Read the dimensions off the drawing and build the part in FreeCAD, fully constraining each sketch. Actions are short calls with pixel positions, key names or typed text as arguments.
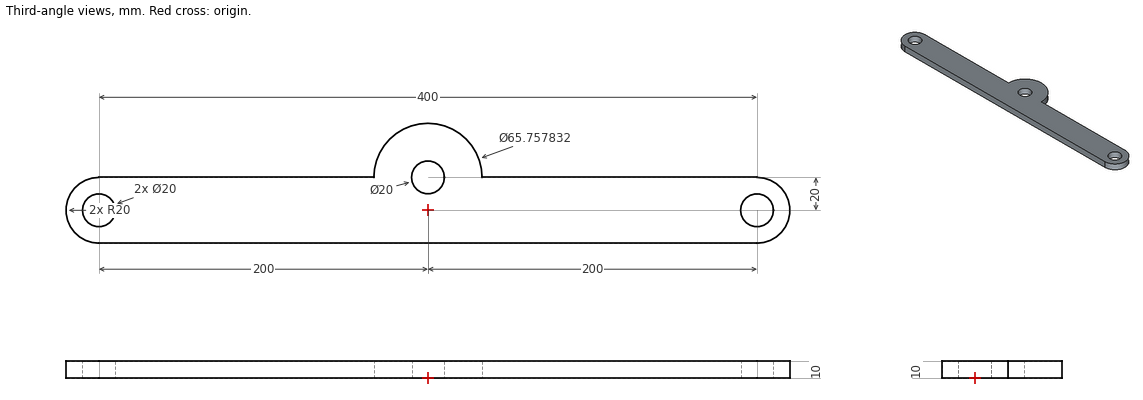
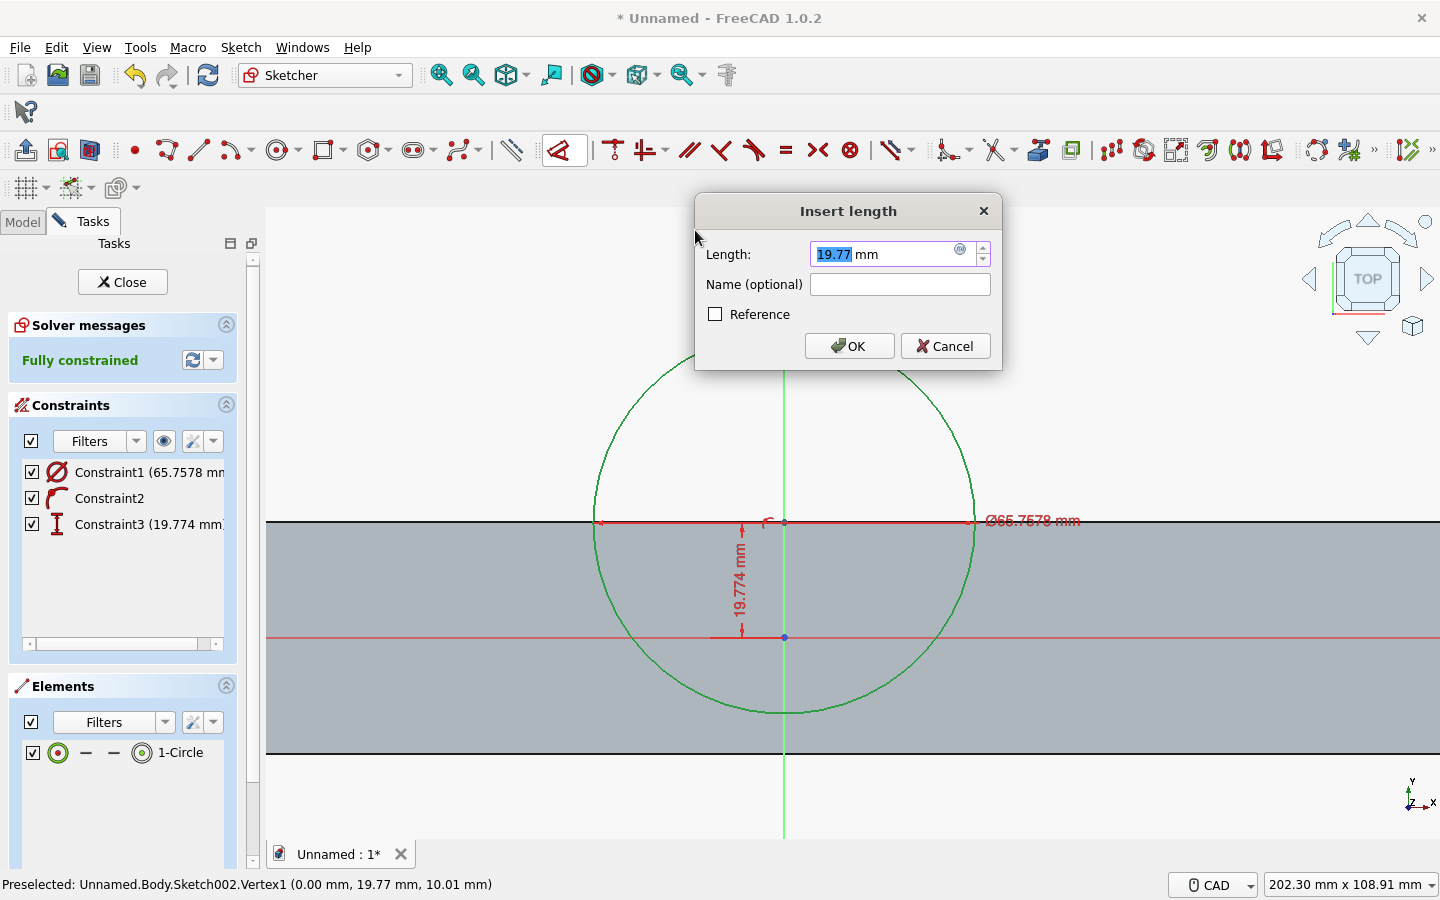
text(20)
key(Return)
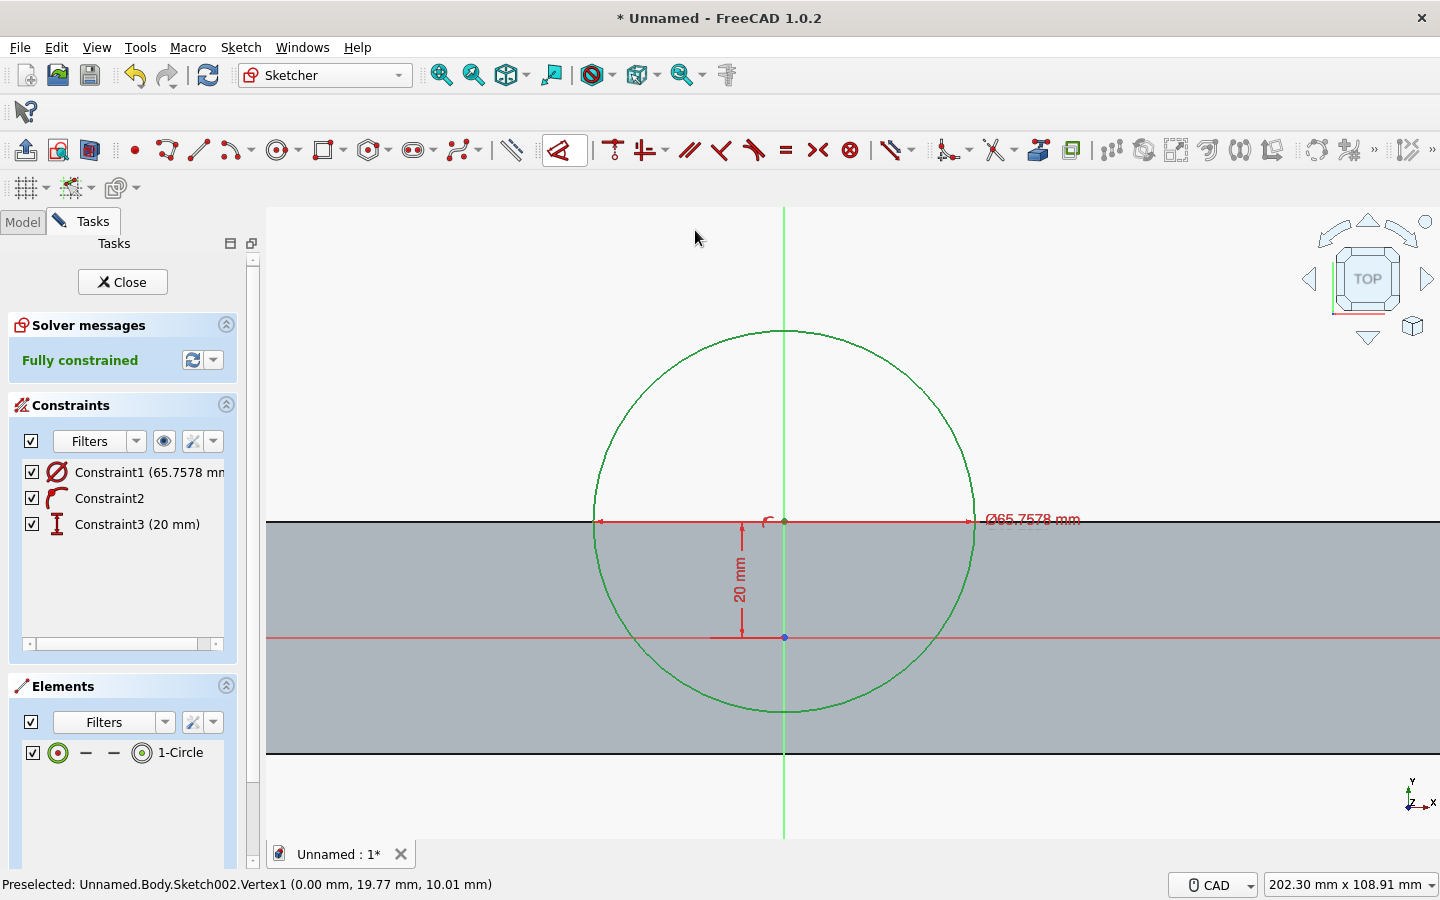
click(123, 282)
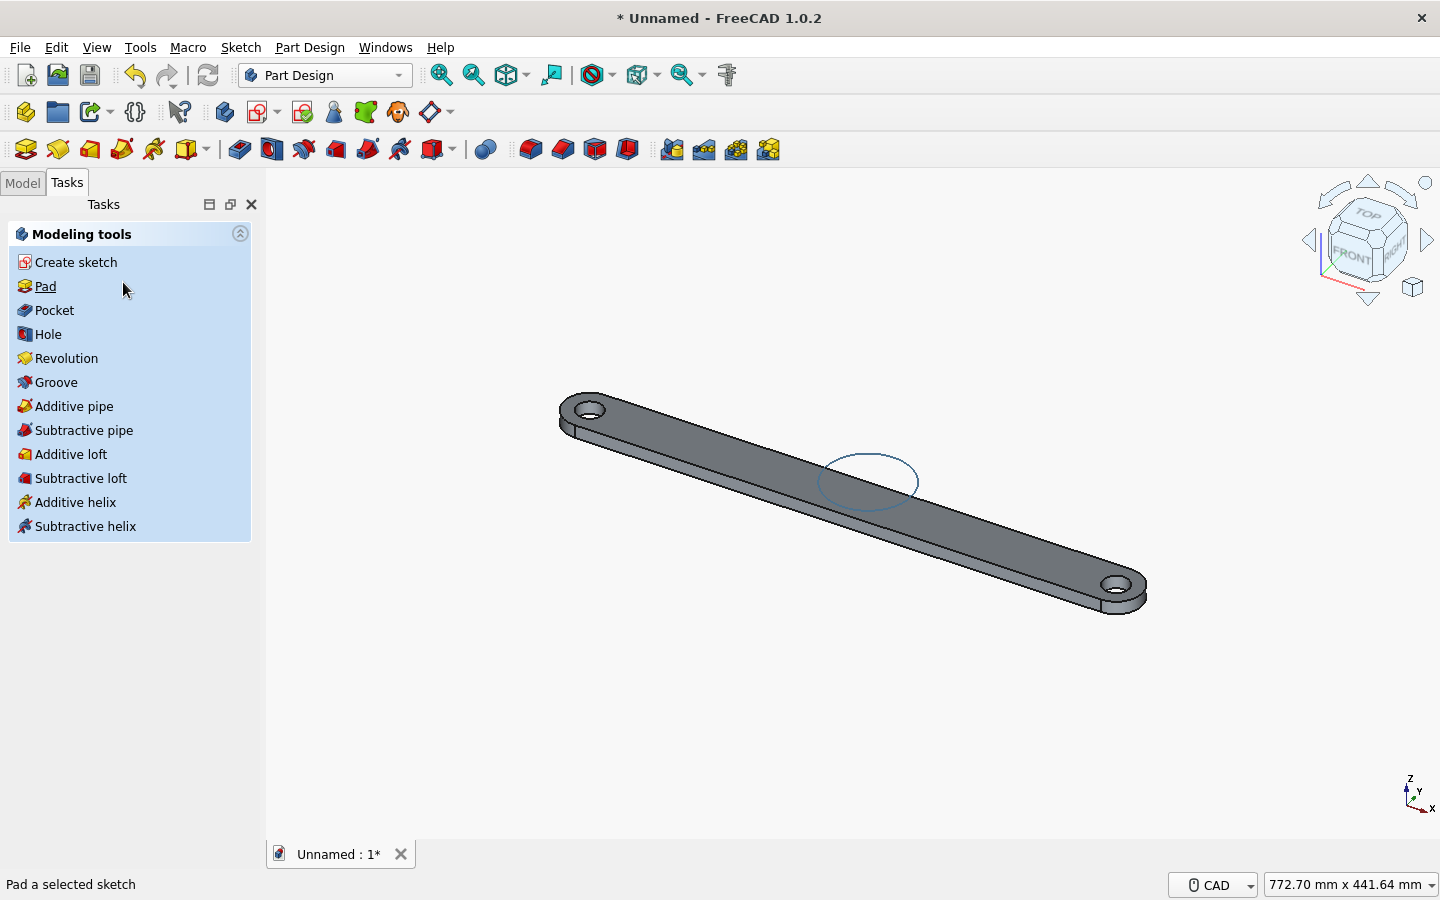
click(26, 150)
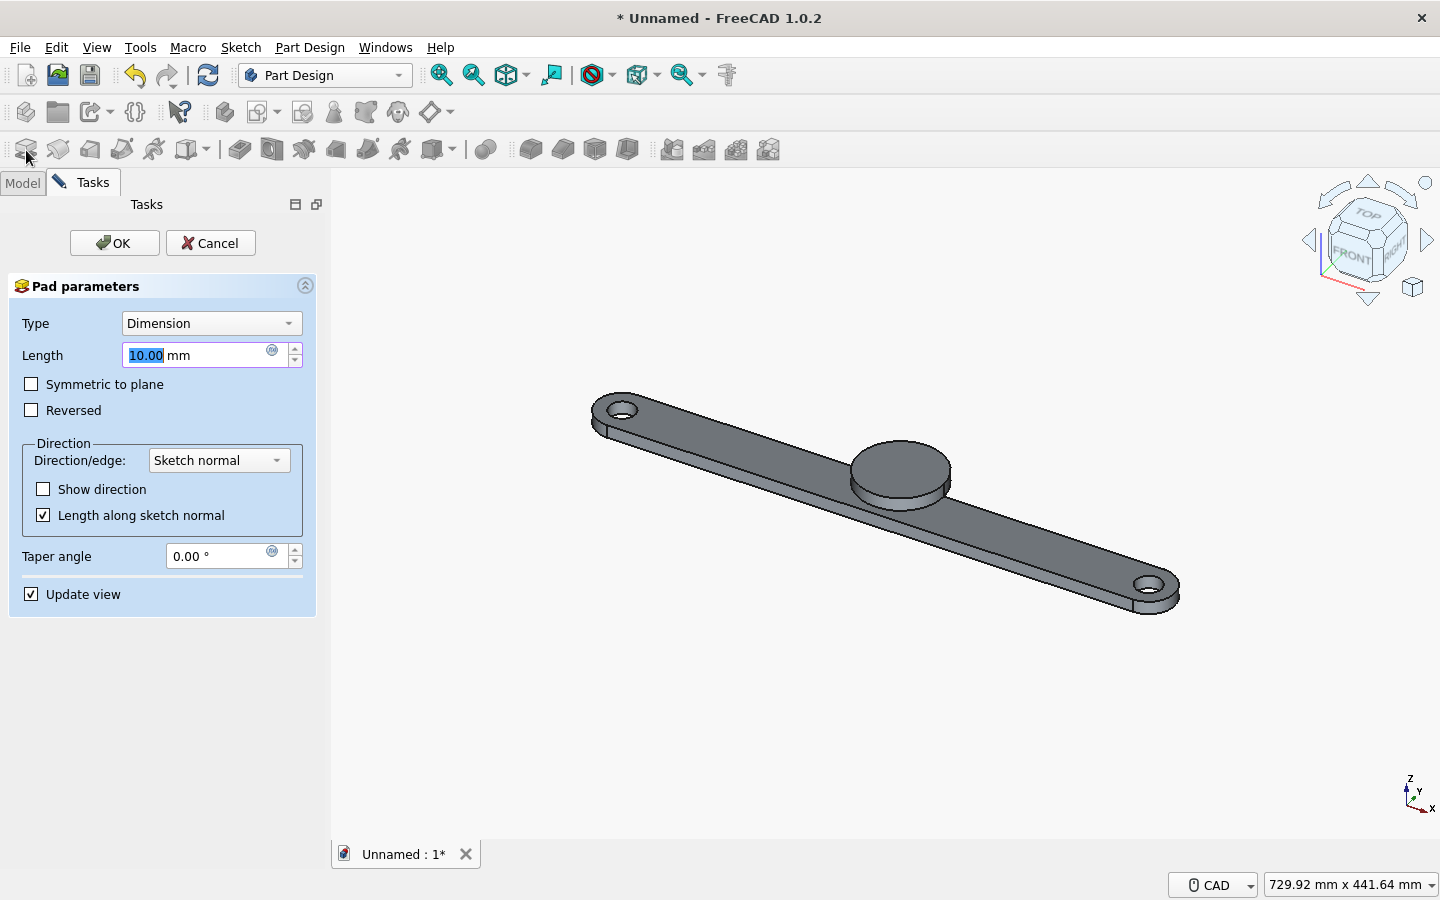
text(10)
key(Tab)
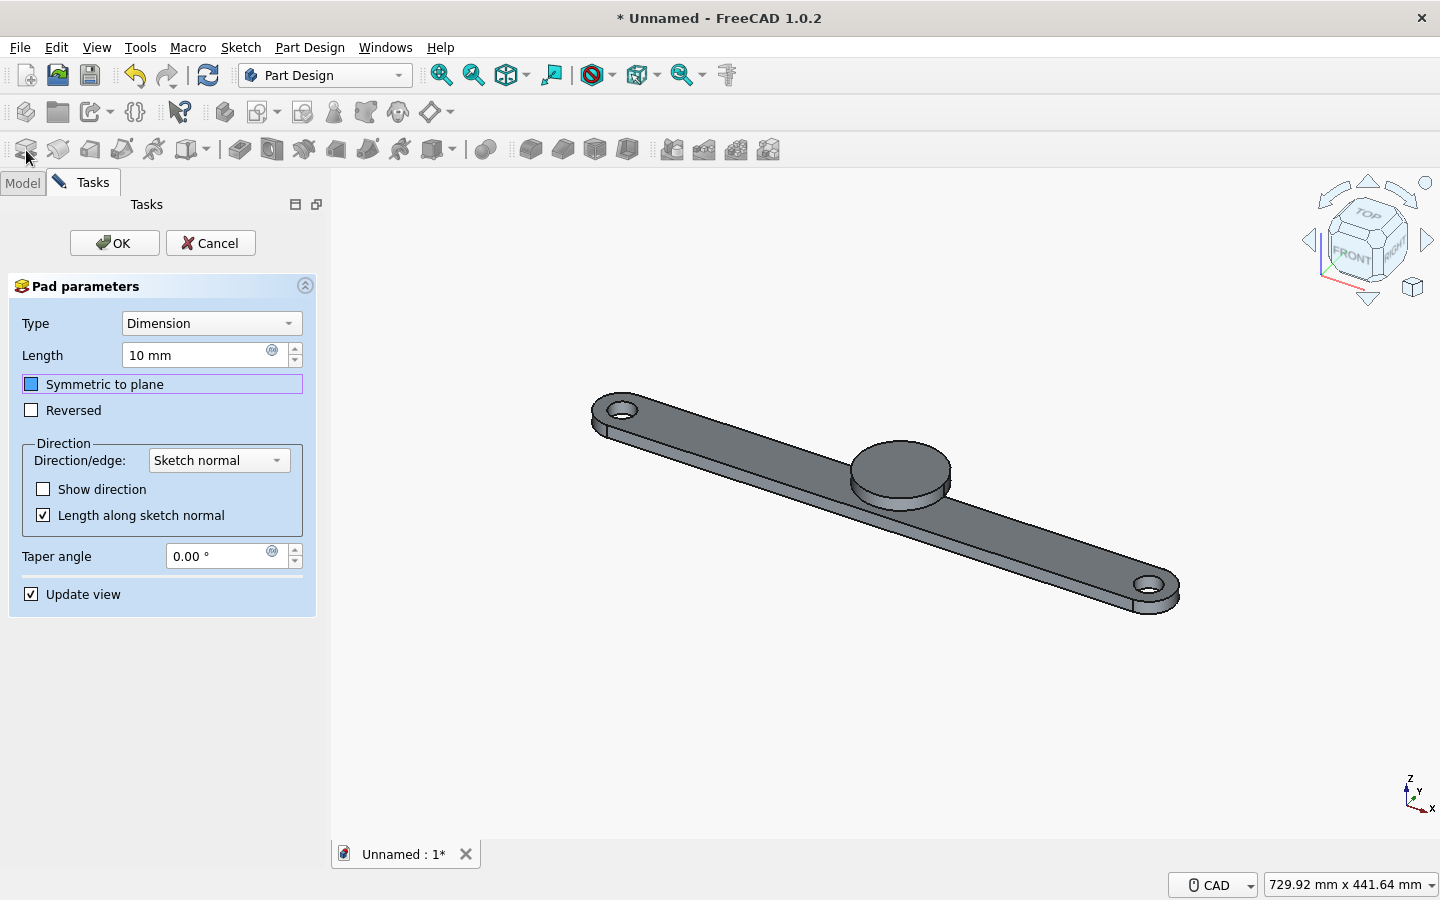
click(30, 410)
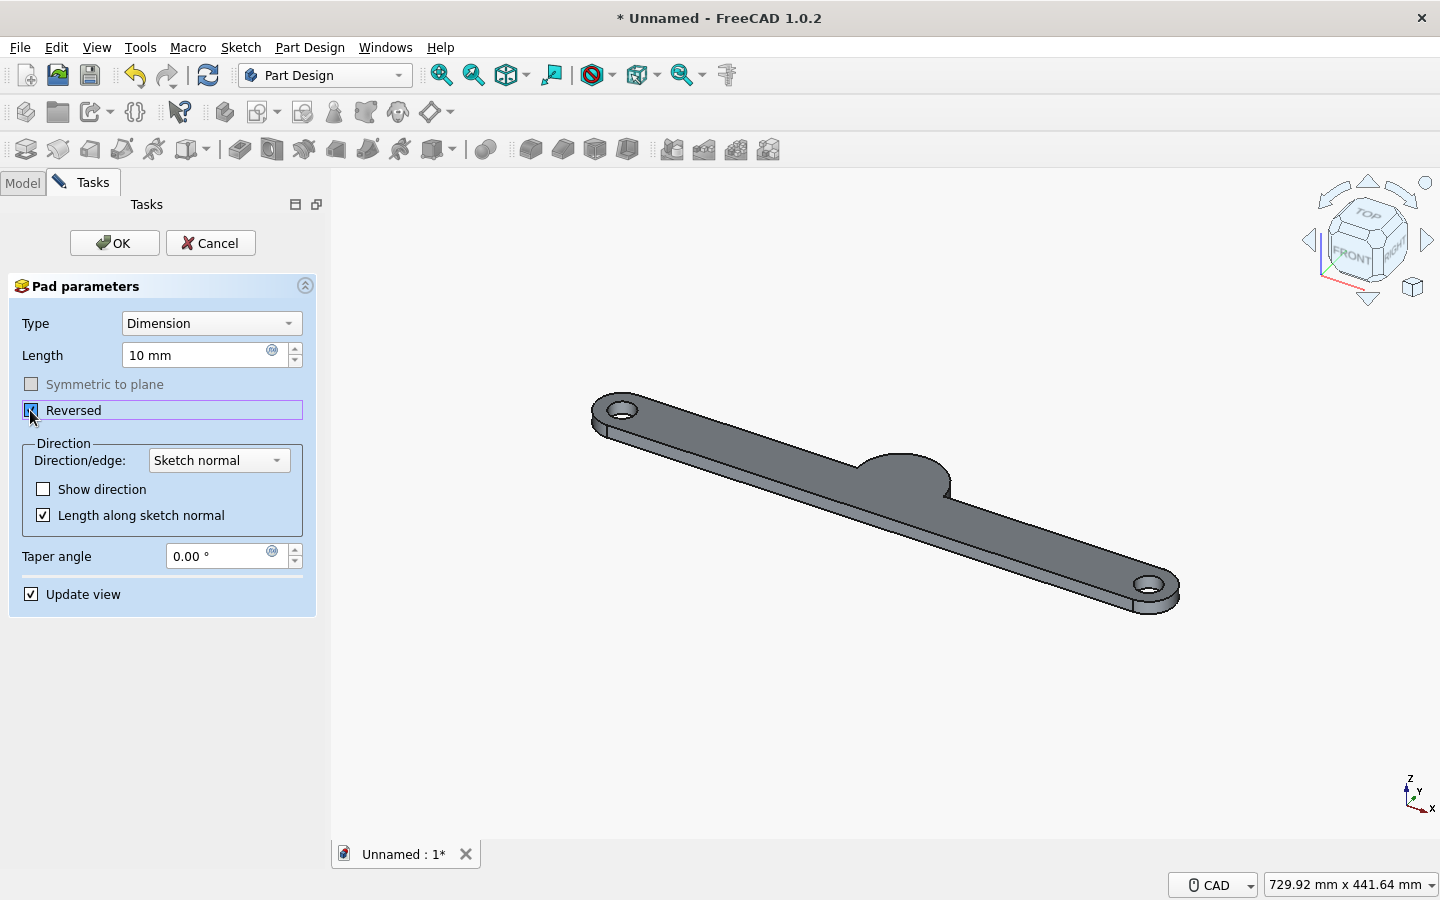
click(115, 243)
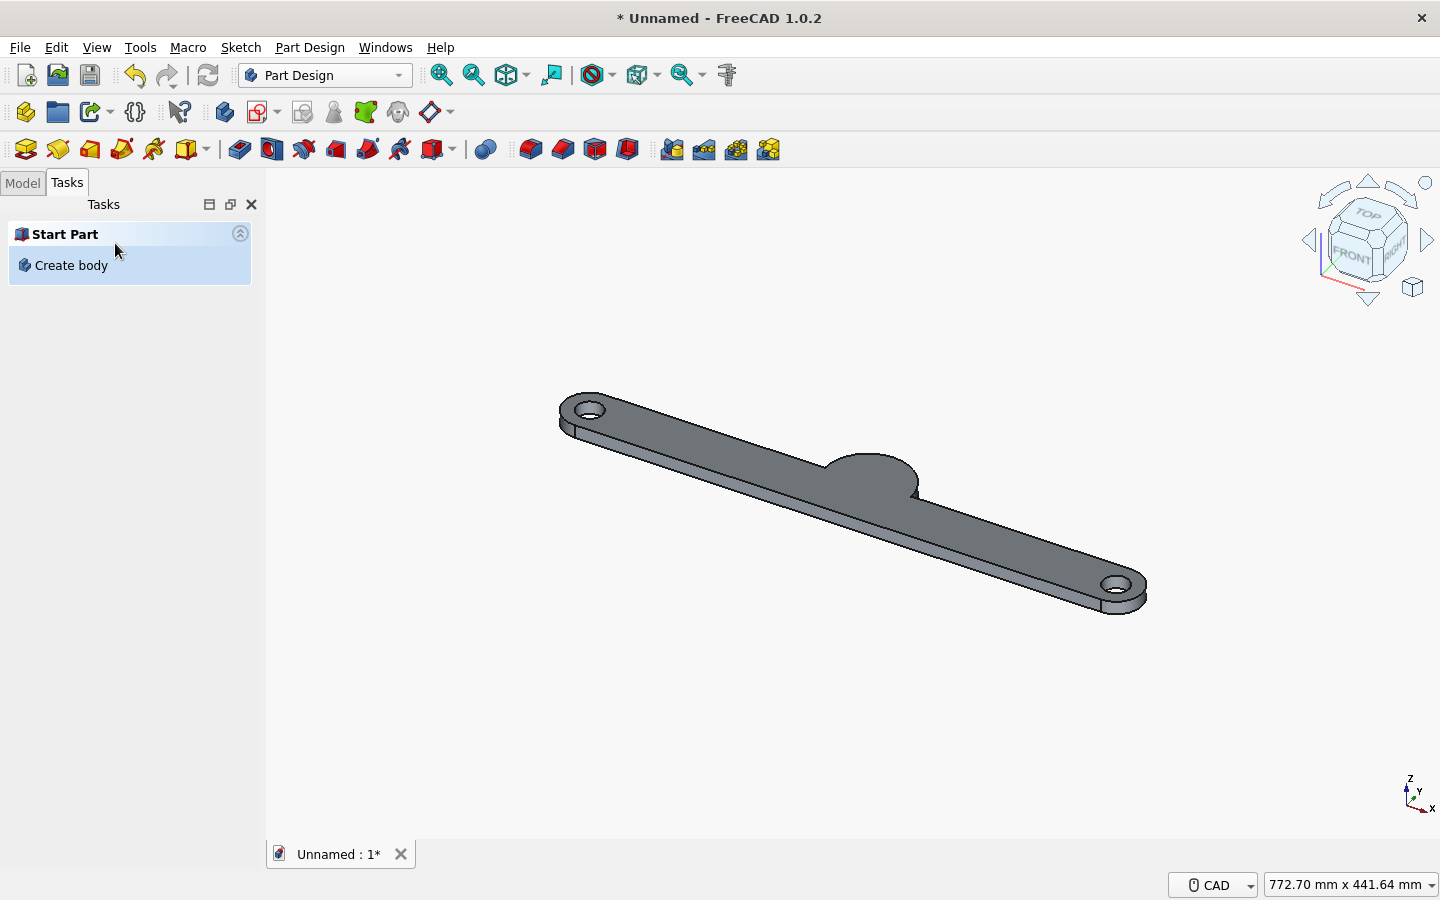
click(865, 484)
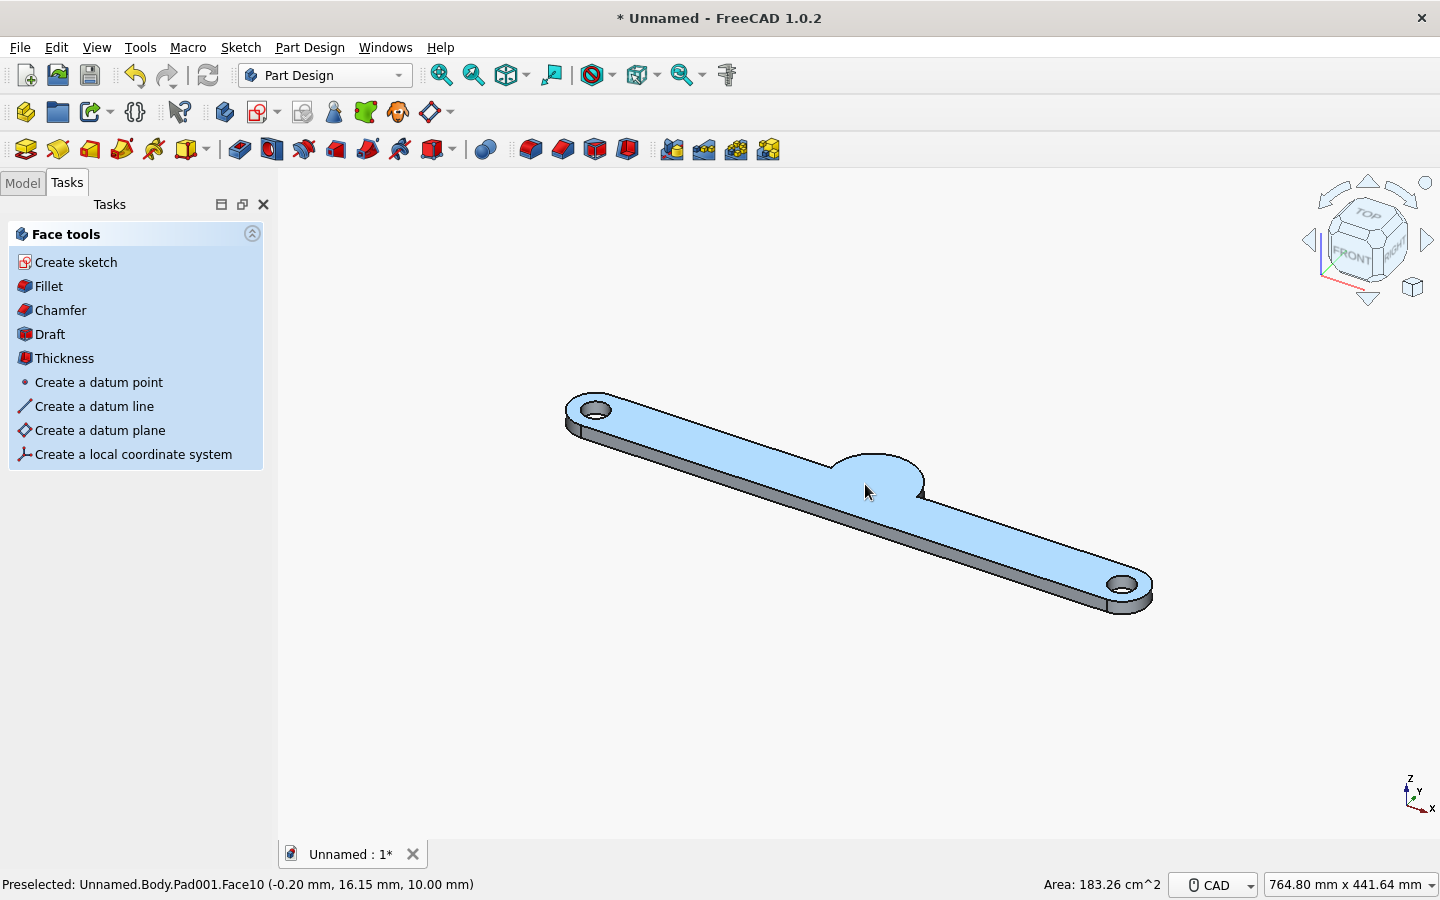
click(258, 112)